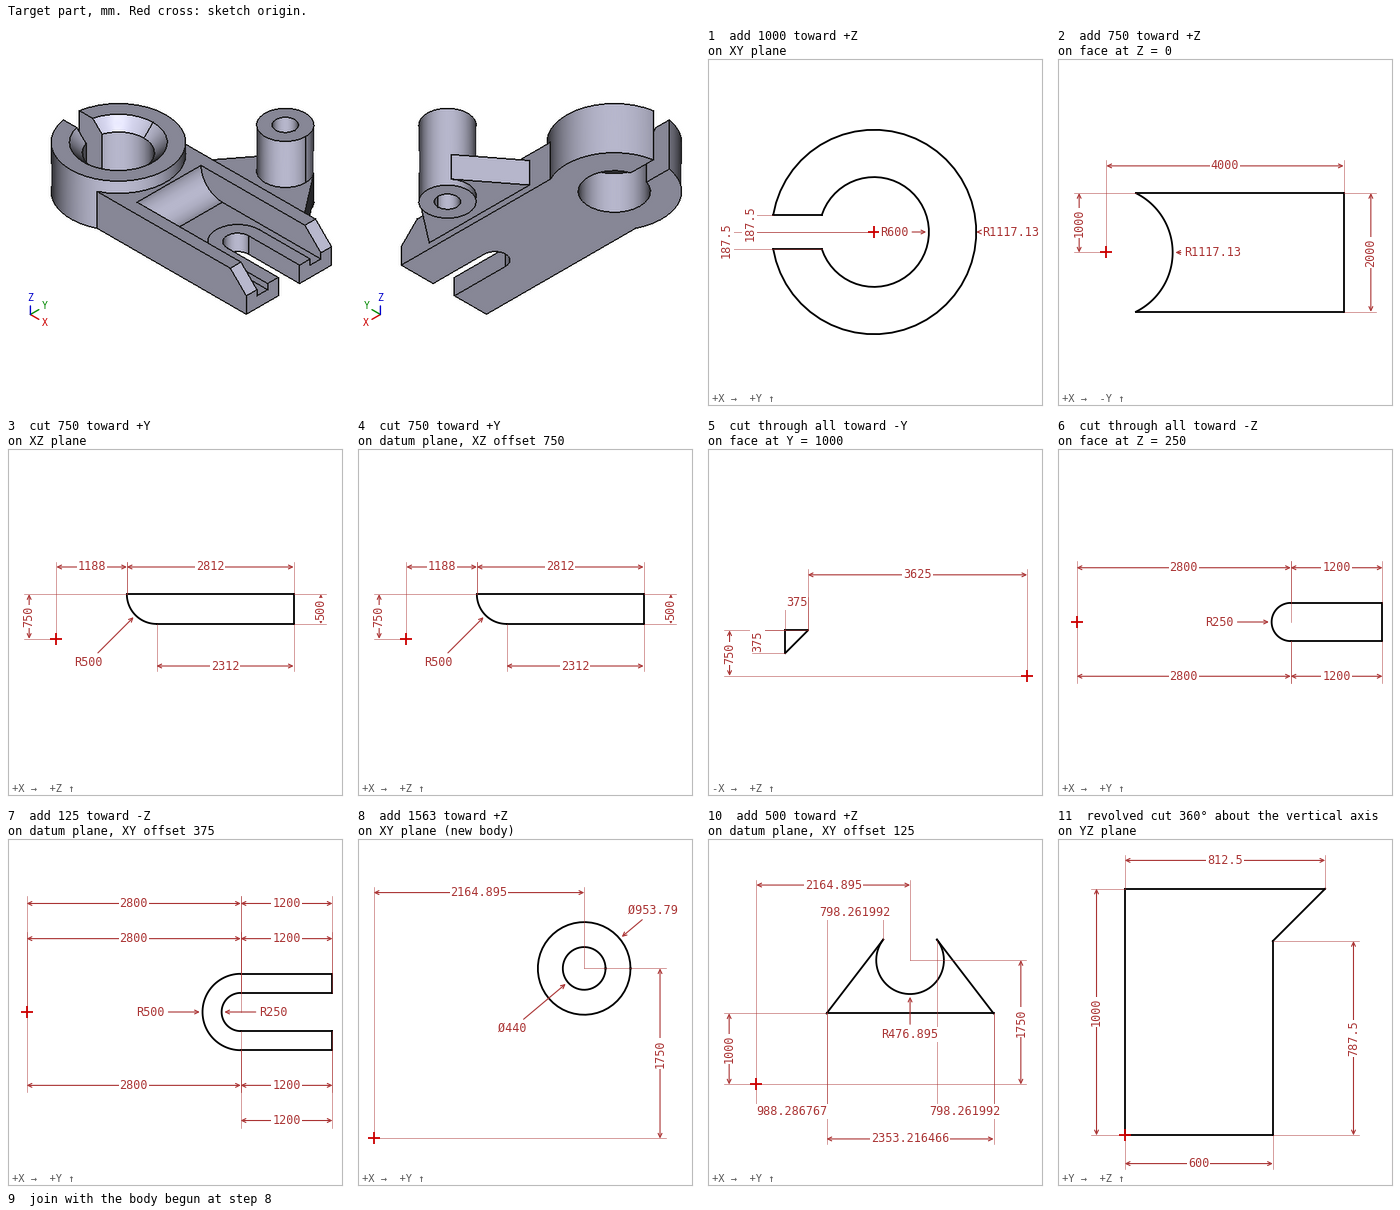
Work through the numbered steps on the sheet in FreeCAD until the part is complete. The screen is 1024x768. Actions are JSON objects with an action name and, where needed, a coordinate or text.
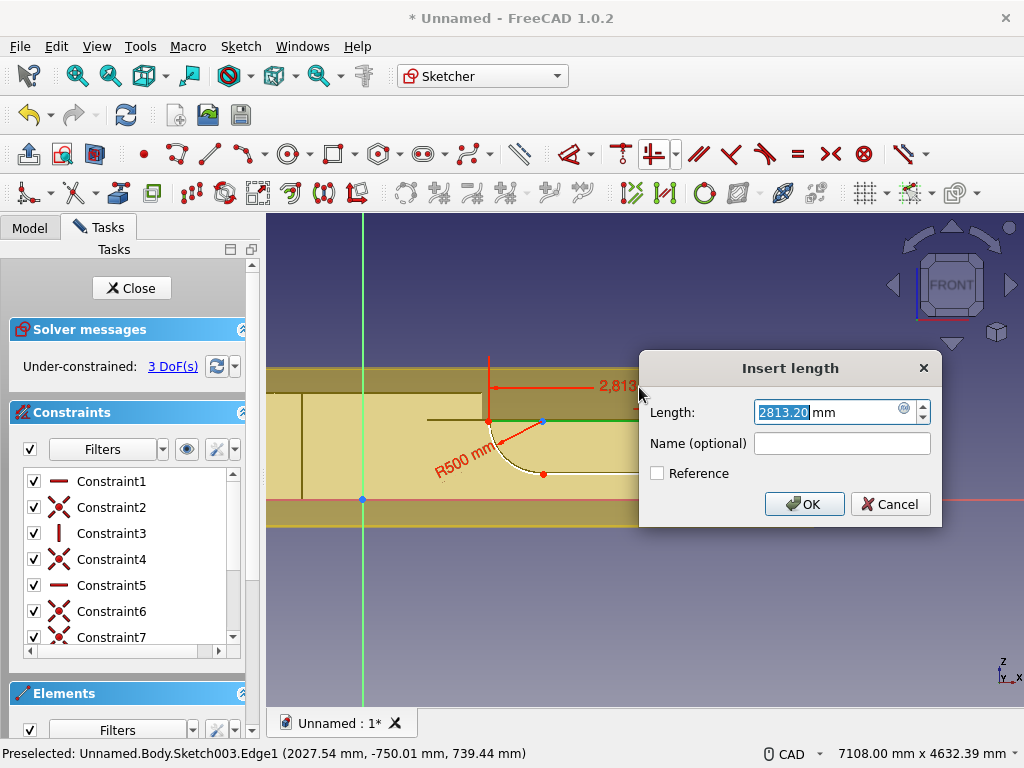
{"action": "type", "text": "2812"}
{"action": "key", "text": "Return"}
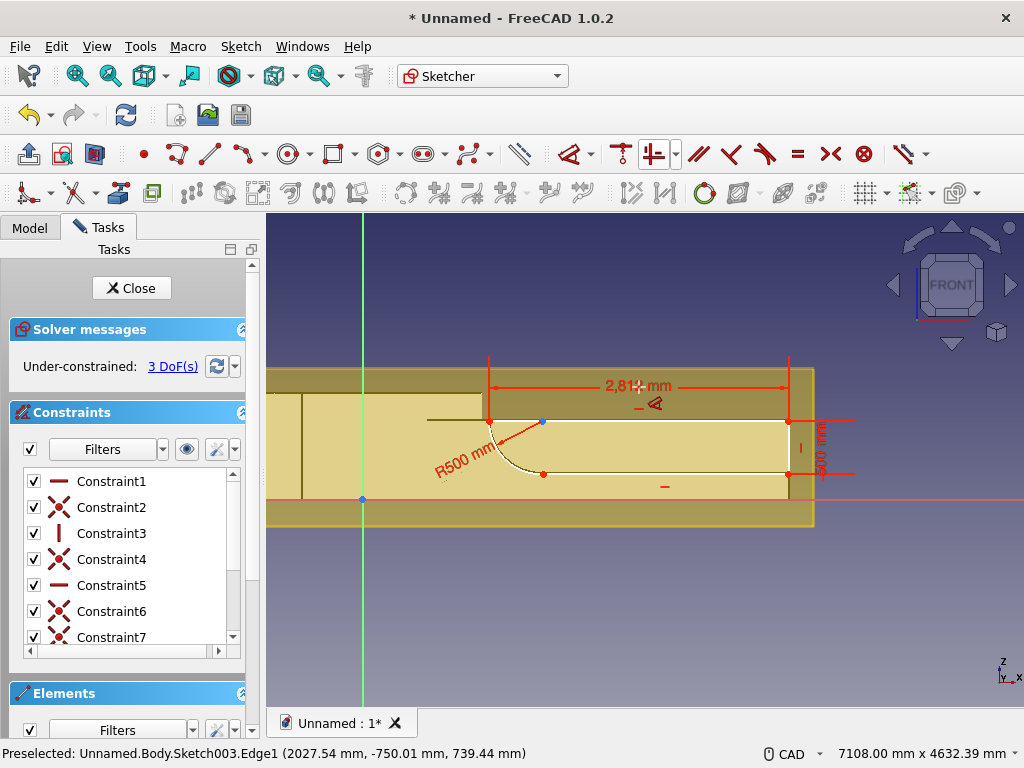
{"action": "left_click", "coordinate": [715, 474]}
{"action": "left_click", "coordinate": [666, 440]}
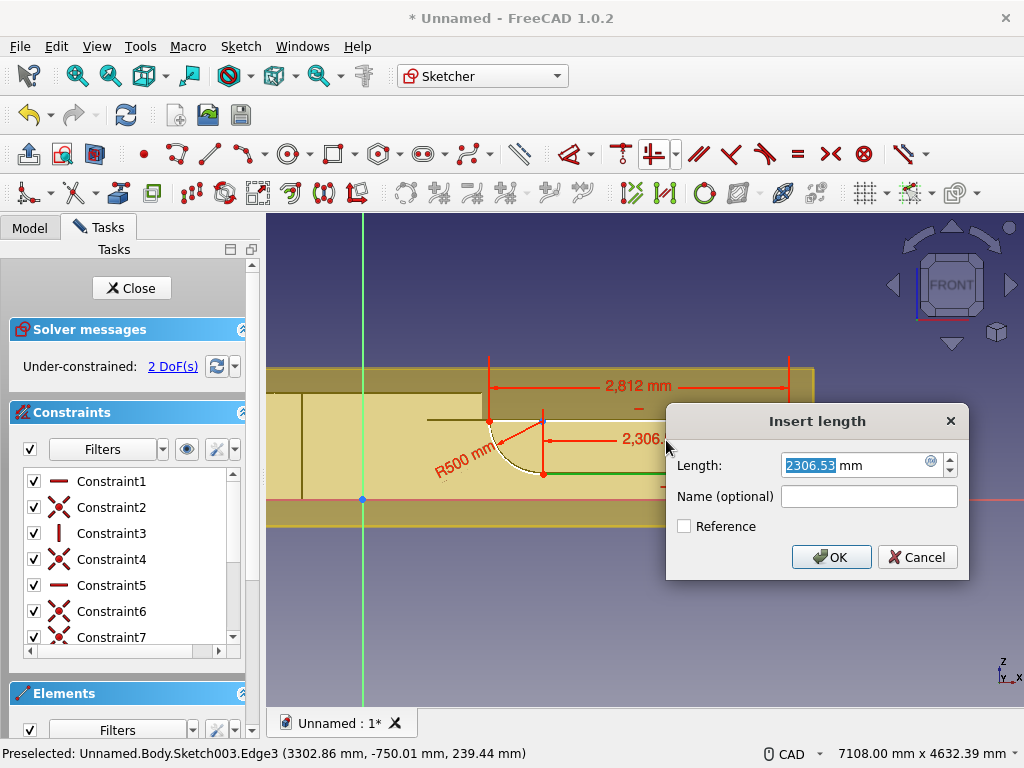
{"action": "type", "text": "2312"}
{"action": "key", "text": "Return"}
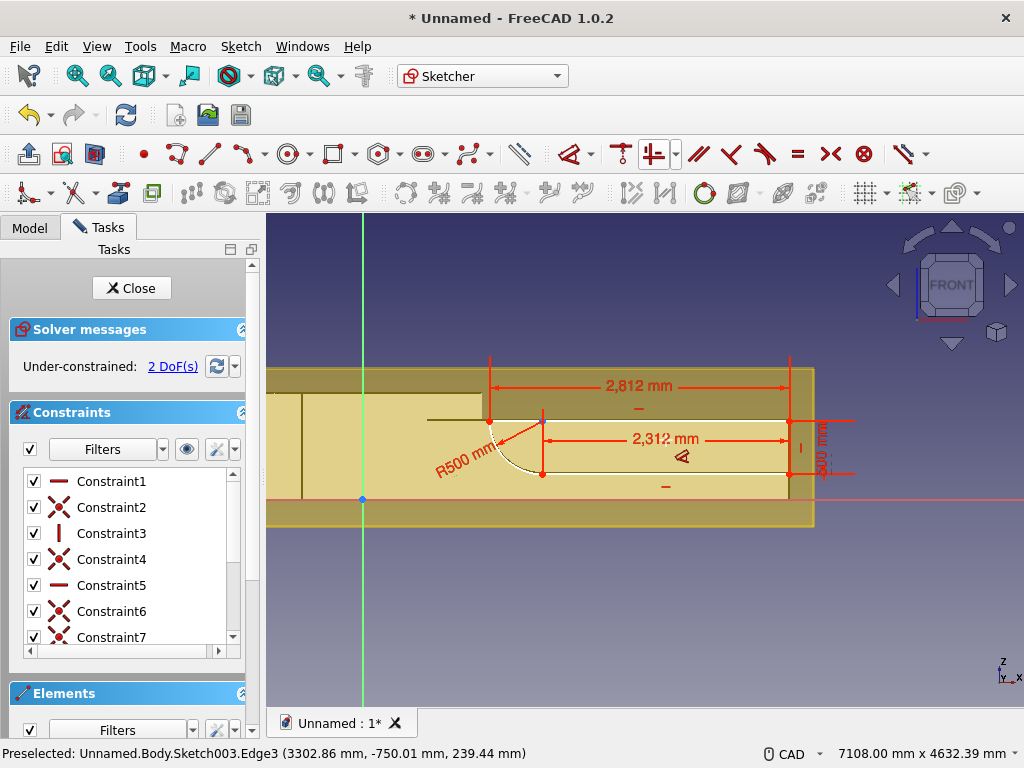
{"action": "left_click", "coordinate": [490, 421]}
{"action": "left_click", "coordinate": [329, 461]}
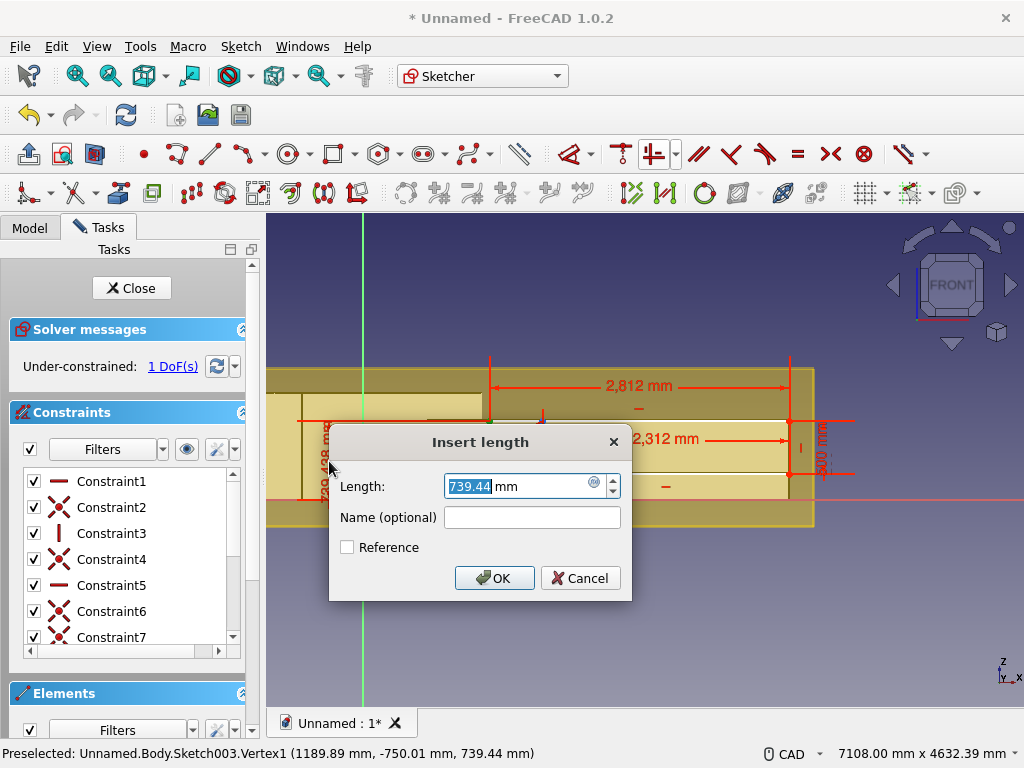
{"action": "type", "text": "750"}
{"action": "key", "text": "Return"}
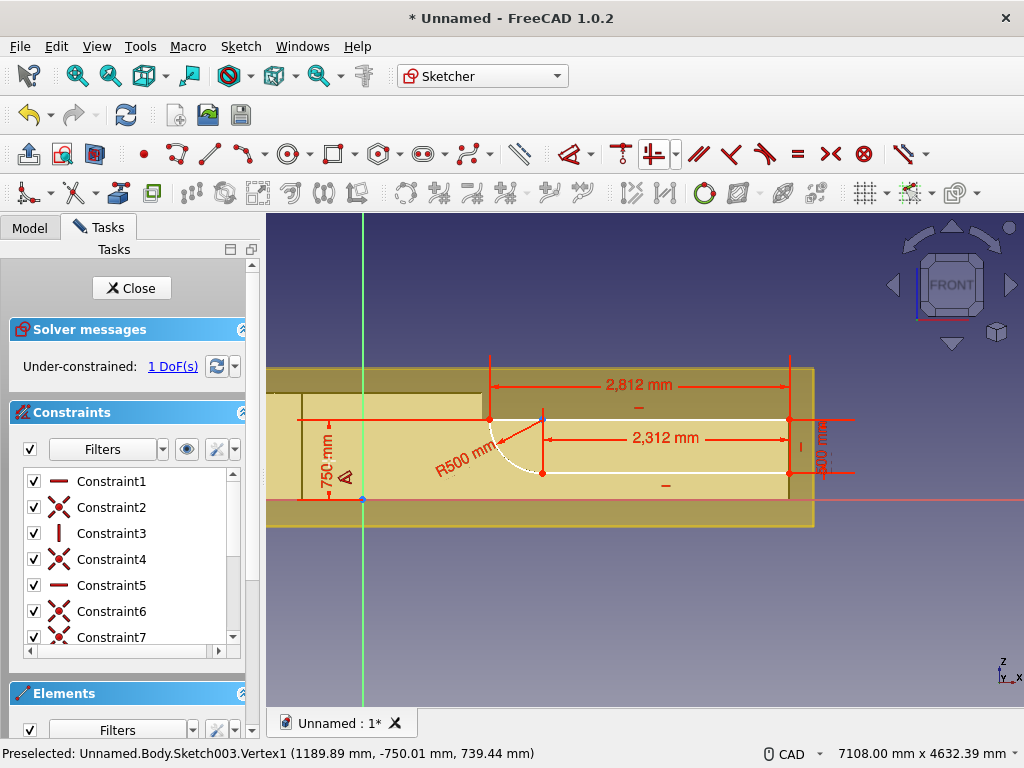
{"action": "left_click", "coordinate": [490, 420]}
{"action": "left_click", "coordinate": [426, 386]}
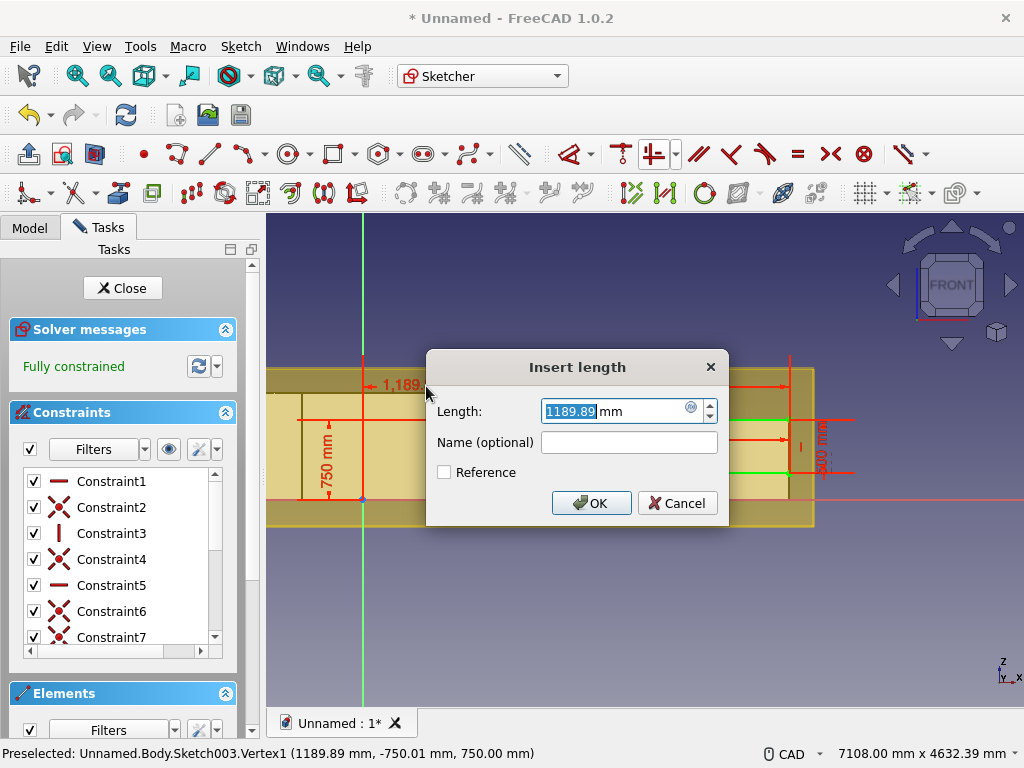
{"action": "type", "text": "1188"}
{"action": "key", "text": "Return"}
{"action": "key", "text": "Escape"}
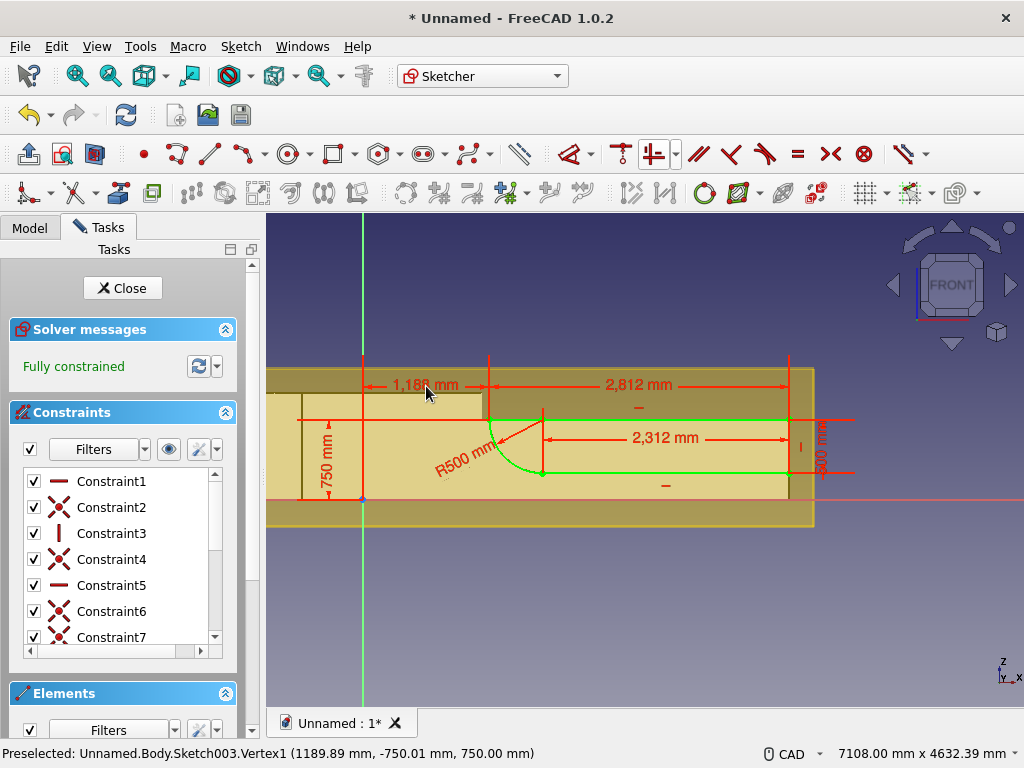
{"action": "left_click", "coordinate": [123, 288]}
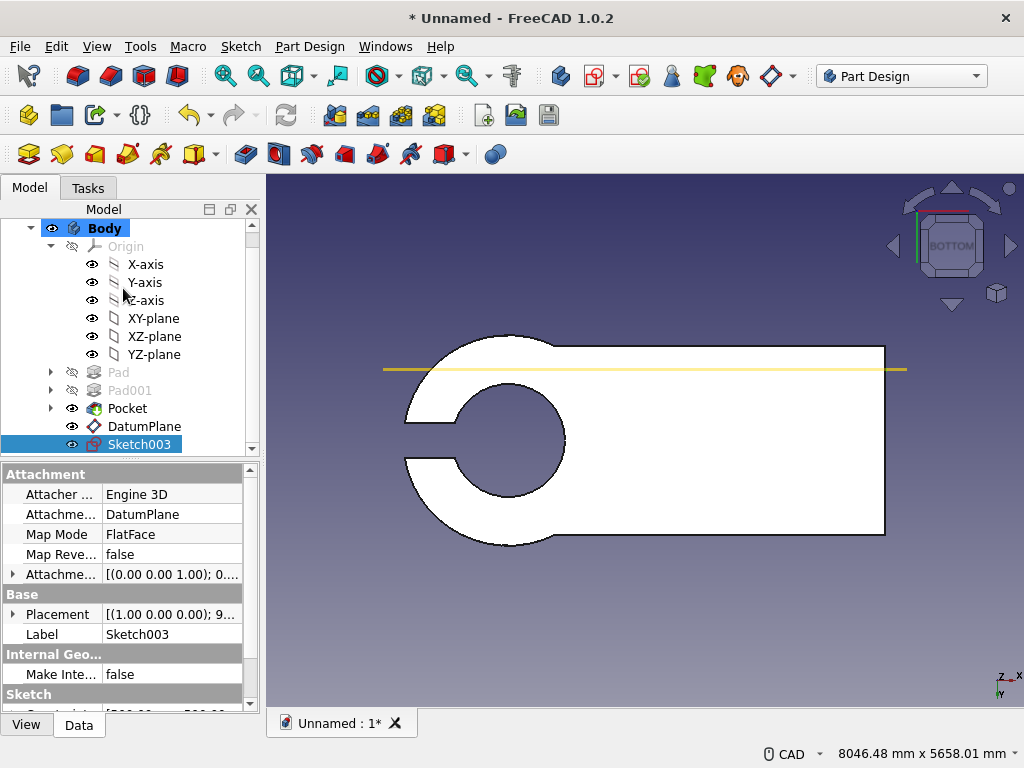
{"action": "left_click", "coordinate": [246, 154]}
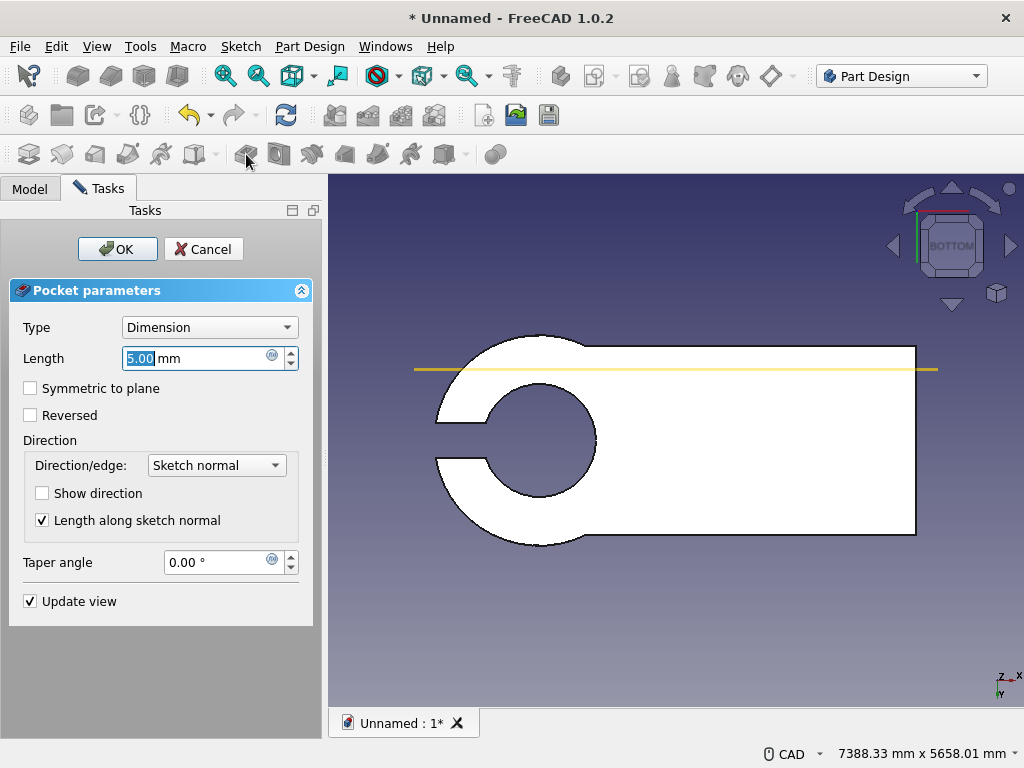
{"action": "type", "text": "750"}
{"action": "key", "text": "Tab"}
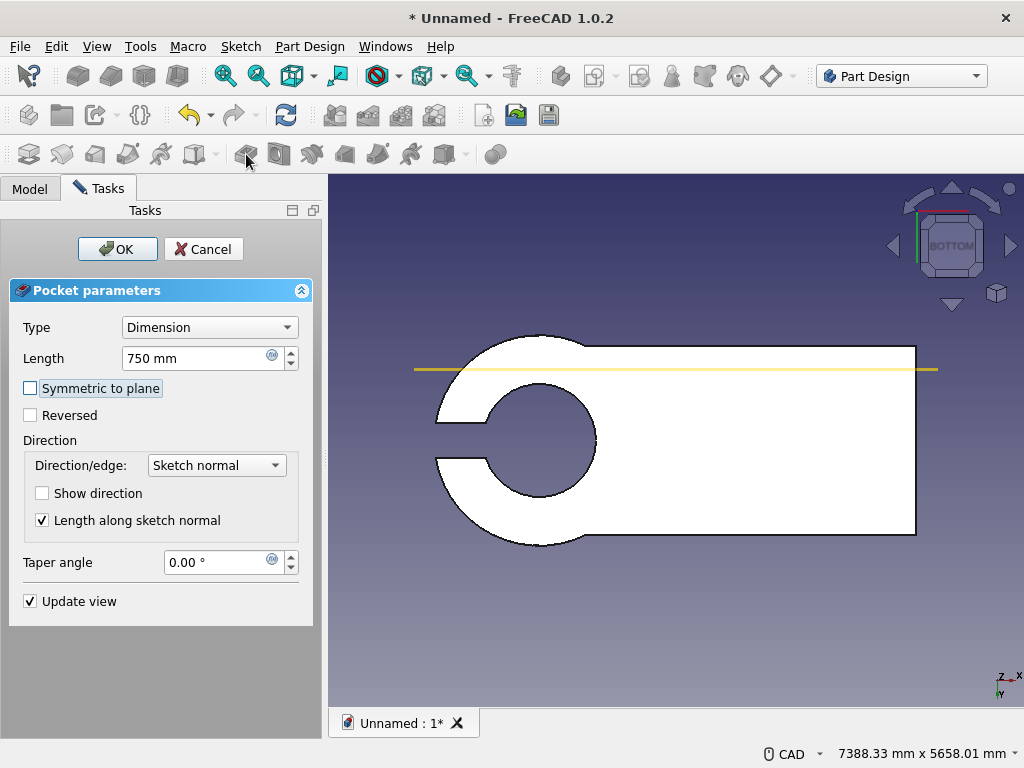
{"action": "left_click", "coordinate": [118, 249]}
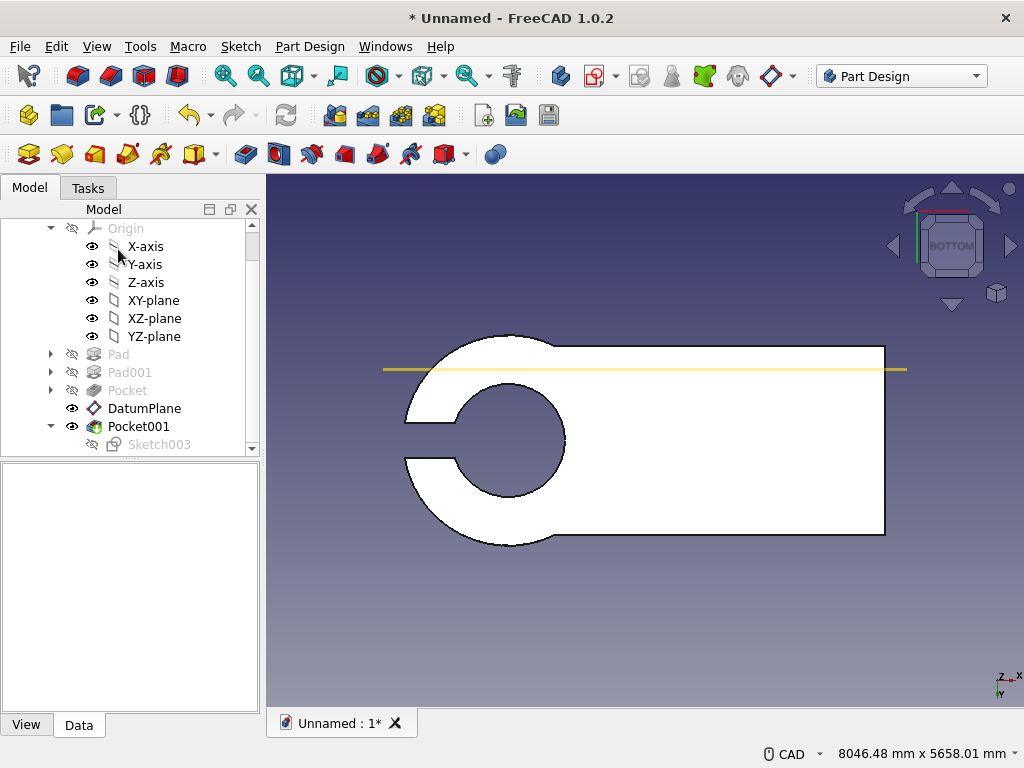
{"action": "left_click", "coordinate": [117, 408]}
{"action": "key", "text": "space"}